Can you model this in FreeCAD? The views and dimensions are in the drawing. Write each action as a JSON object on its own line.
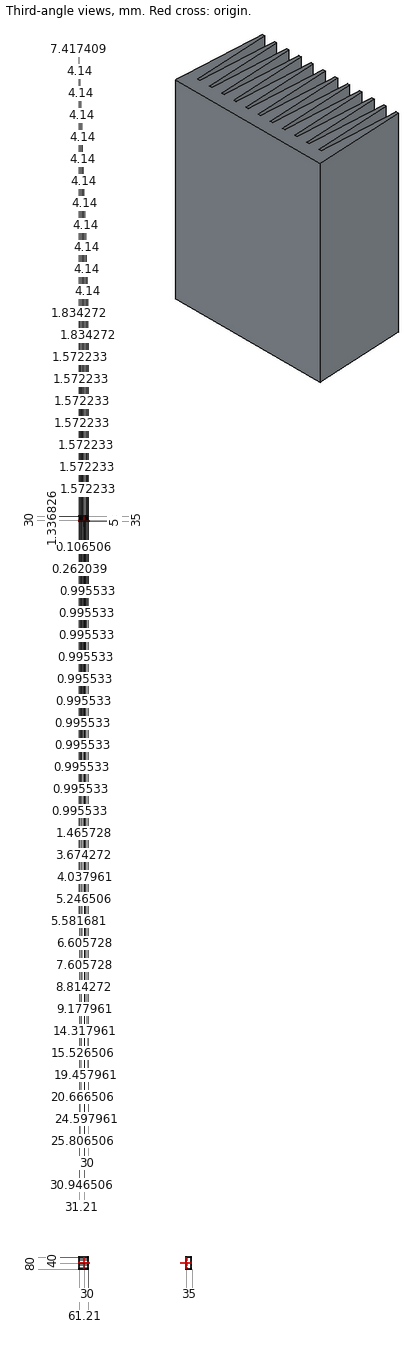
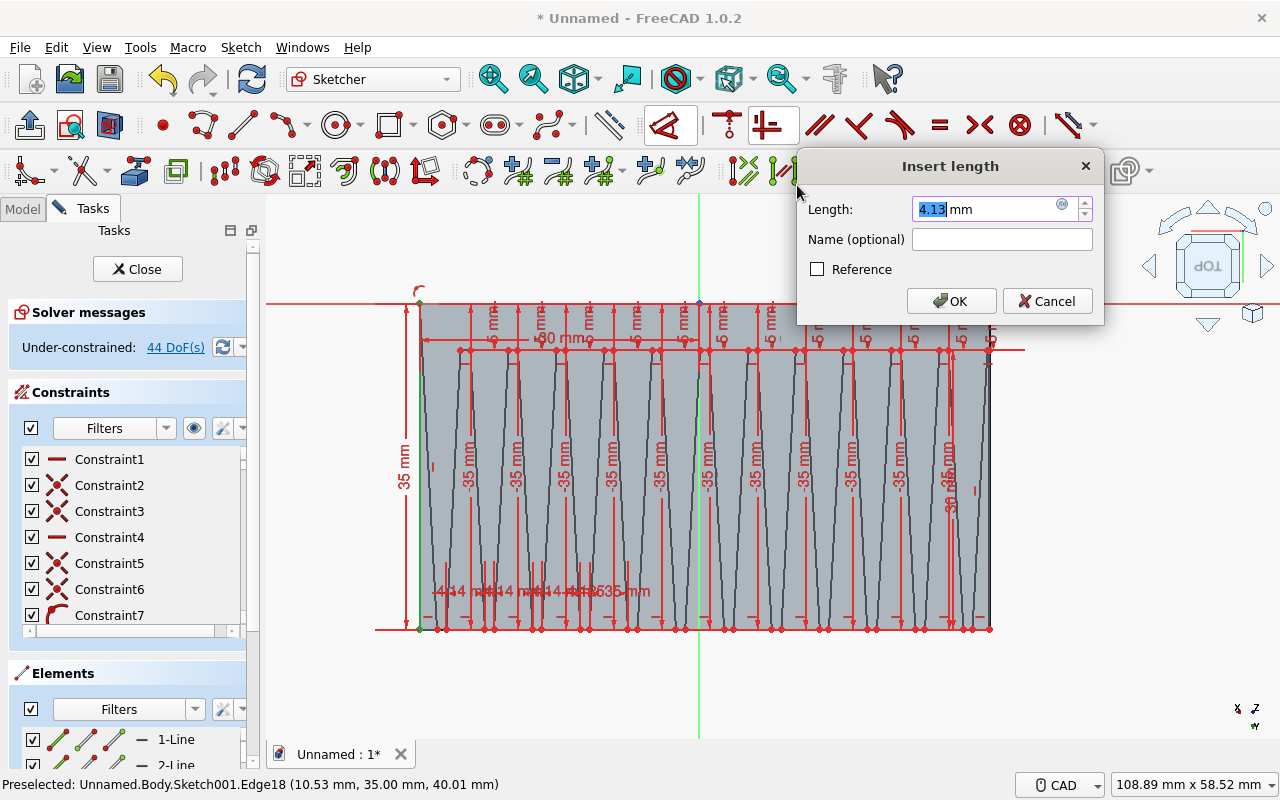
{"action": "type", "text": "4.14"}
{"action": "key", "text": "Return"}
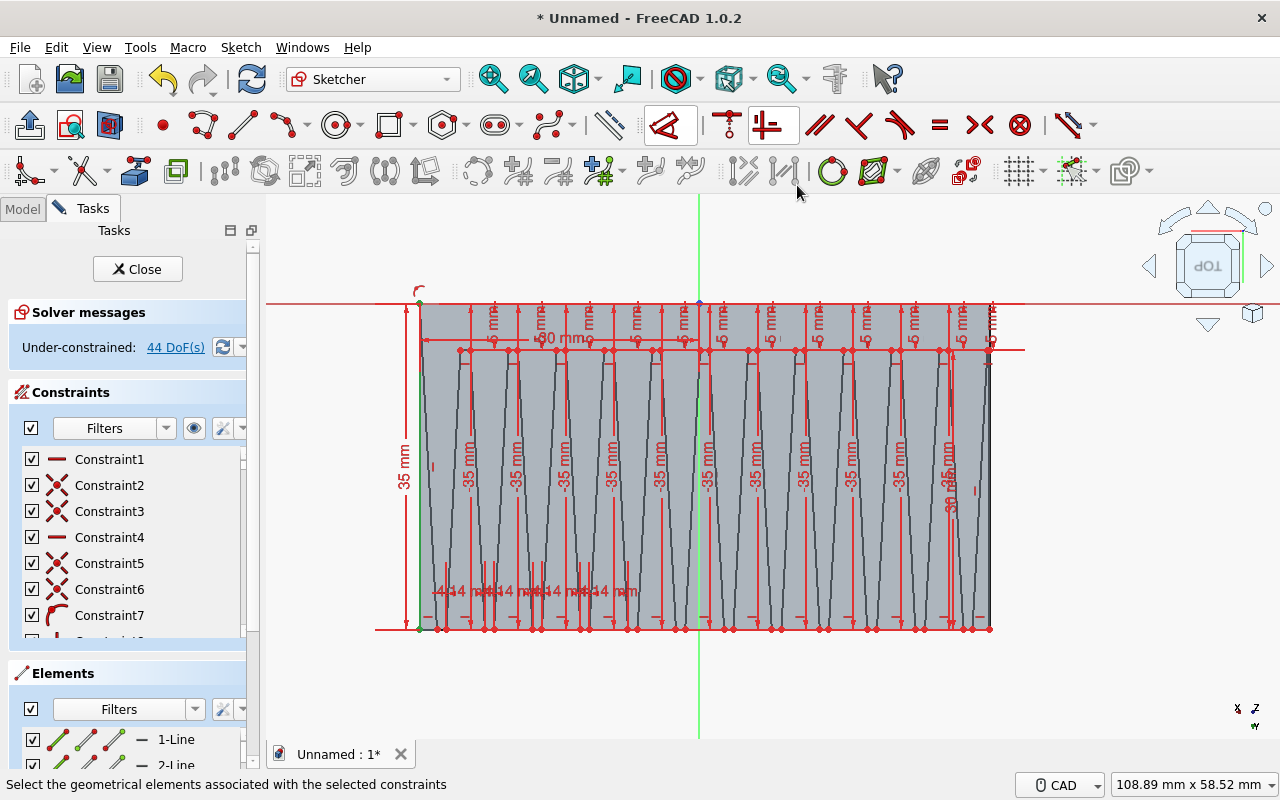
{"action": "left_click", "coordinate": [649, 630]}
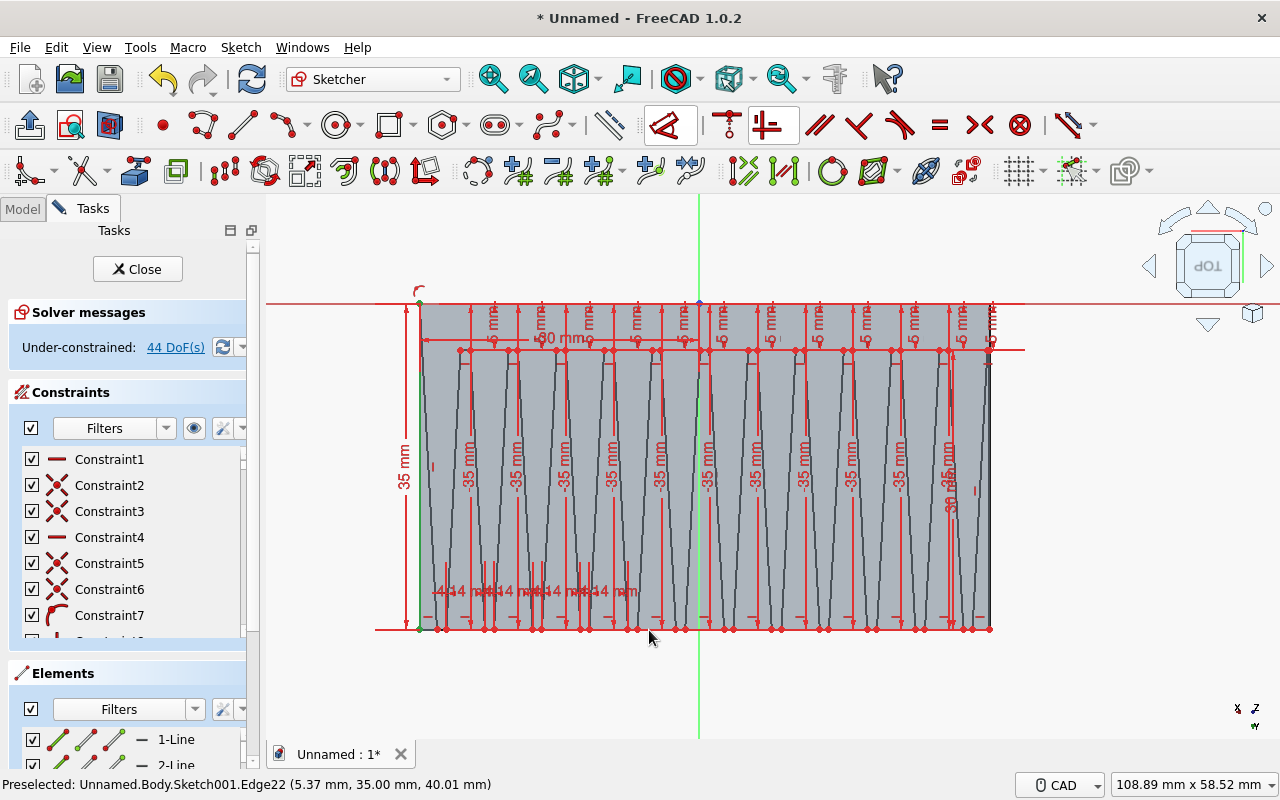
{"action": "key", "text": "l"}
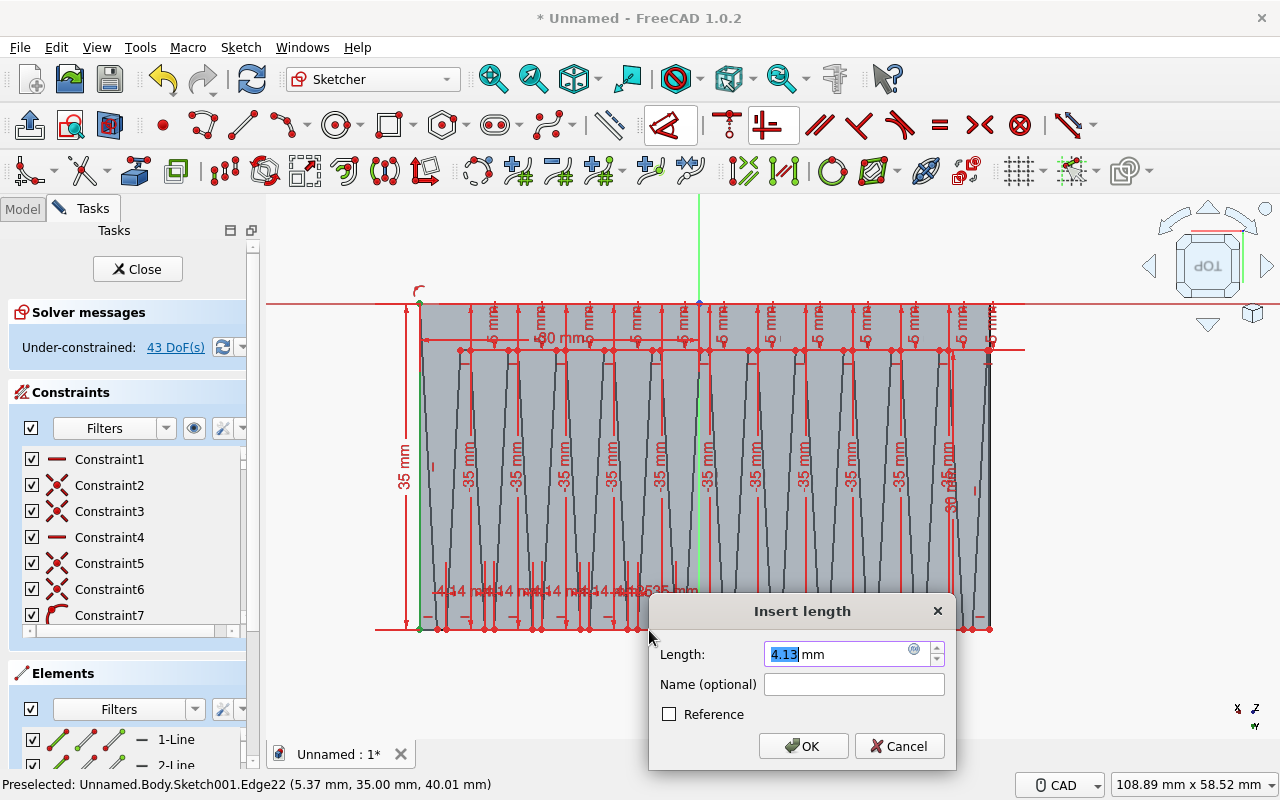
{"action": "type", "text": "4.14"}
{"action": "key", "text": "Return"}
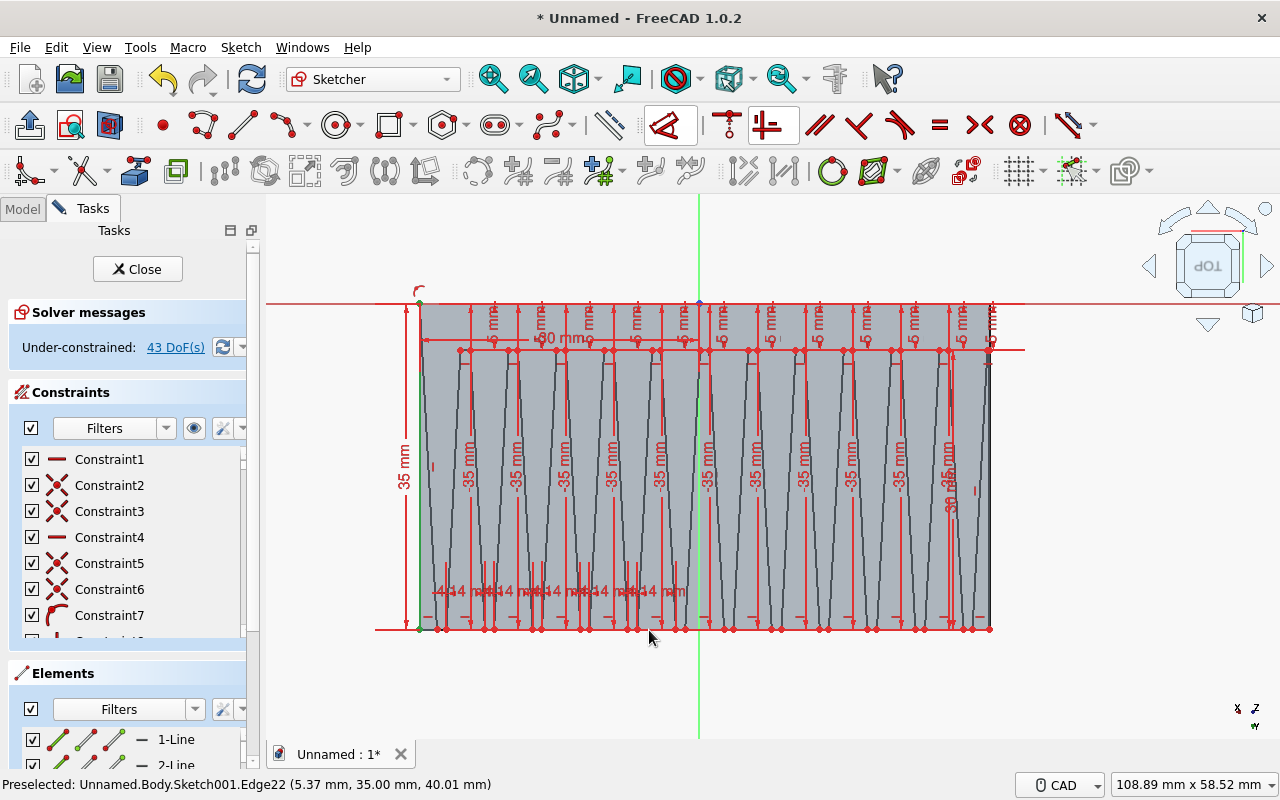
{"action": "left_click", "coordinate": [697, 630]}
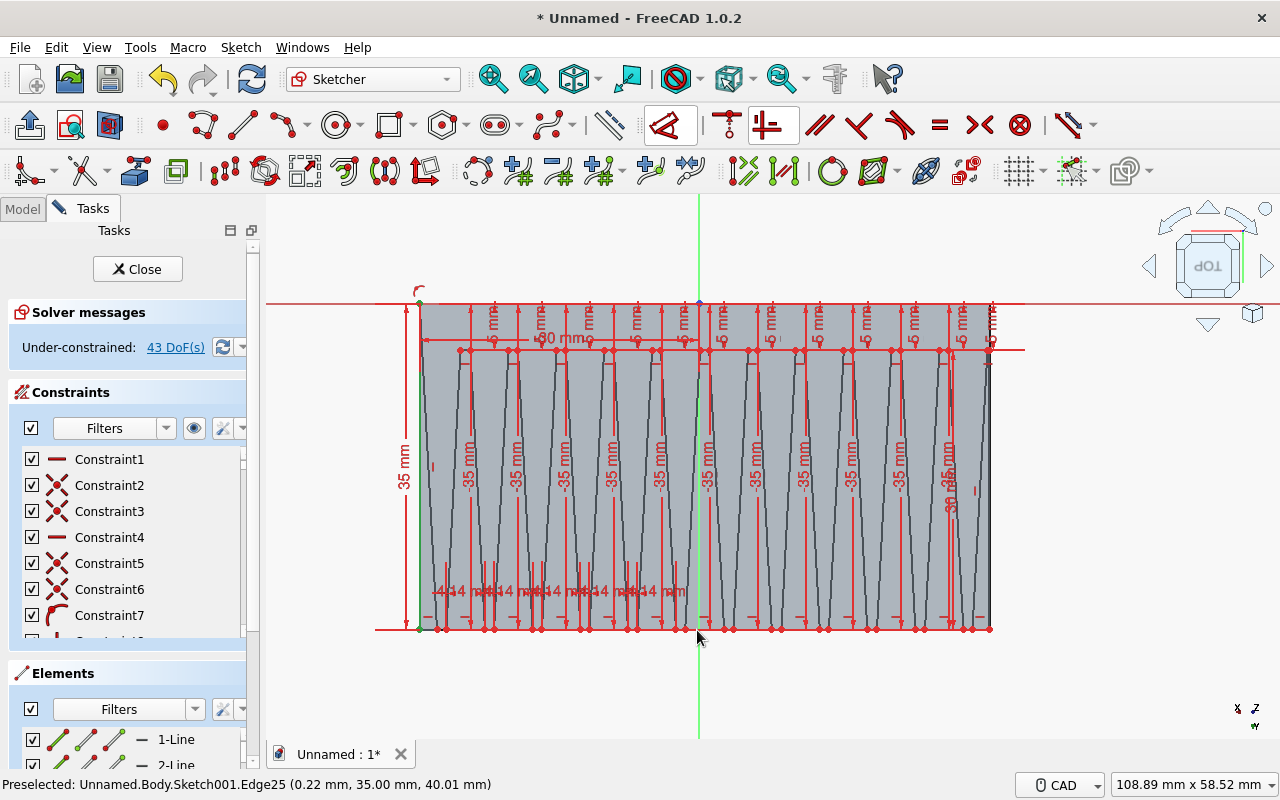
{"action": "left_click", "coordinate": [692, 126]}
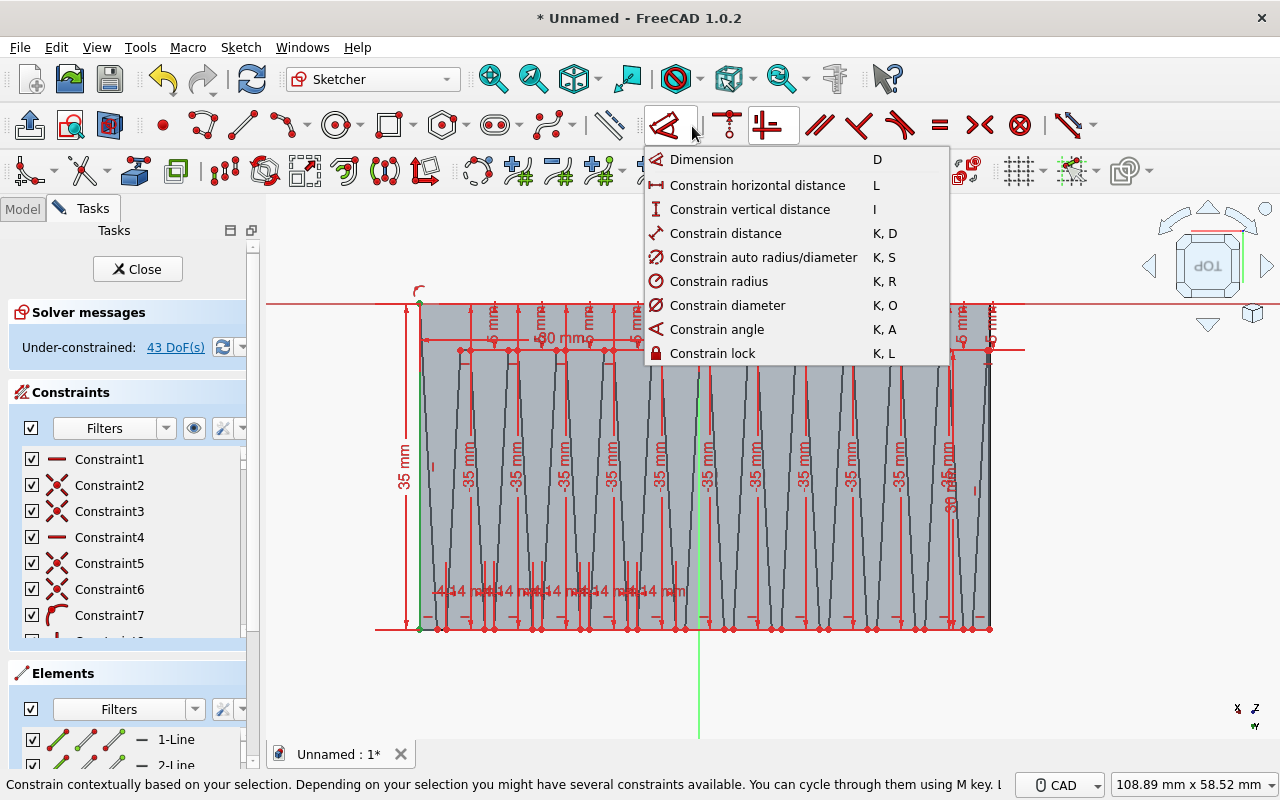
{"action": "left_click", "coordinate": [797, 185]}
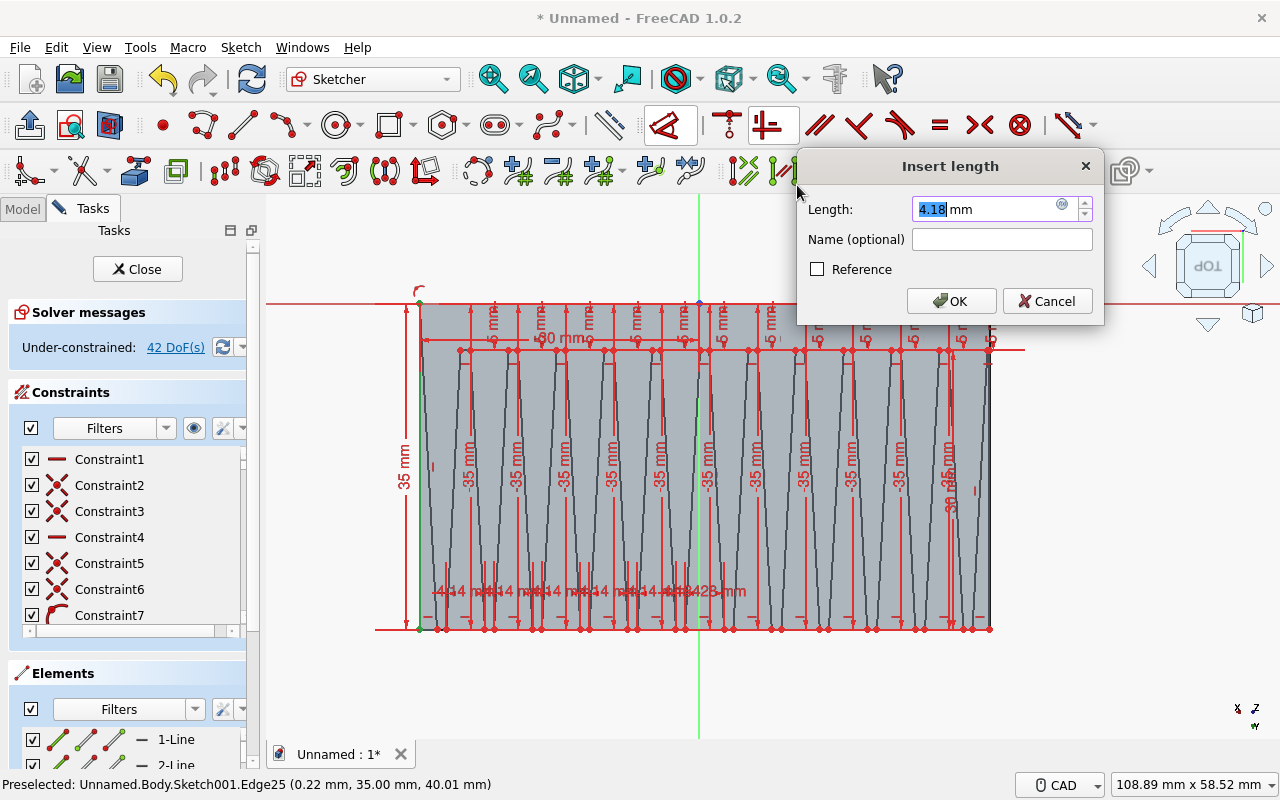
{"action": "type", "text": "4.14"}
{"action": "key", "text": "Return"}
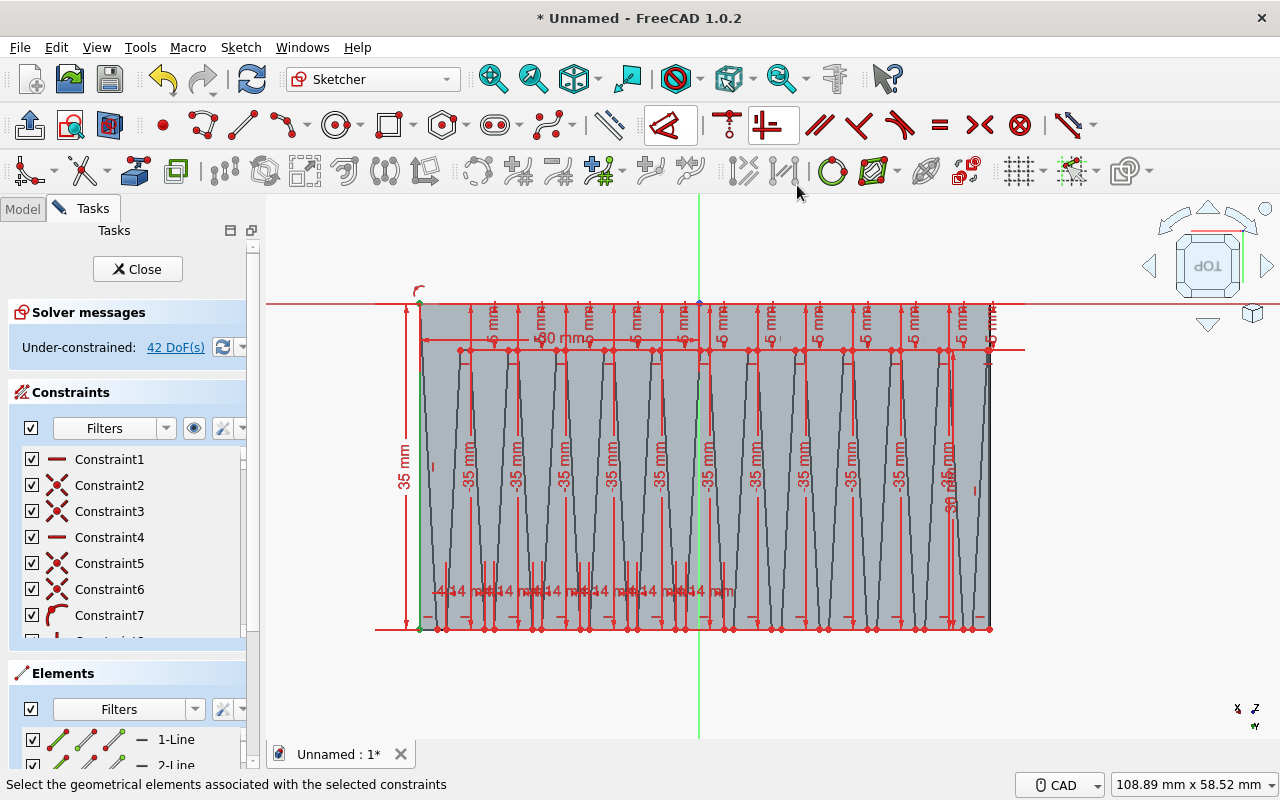
{"action": "left_click", "coordinate": [745, 630]}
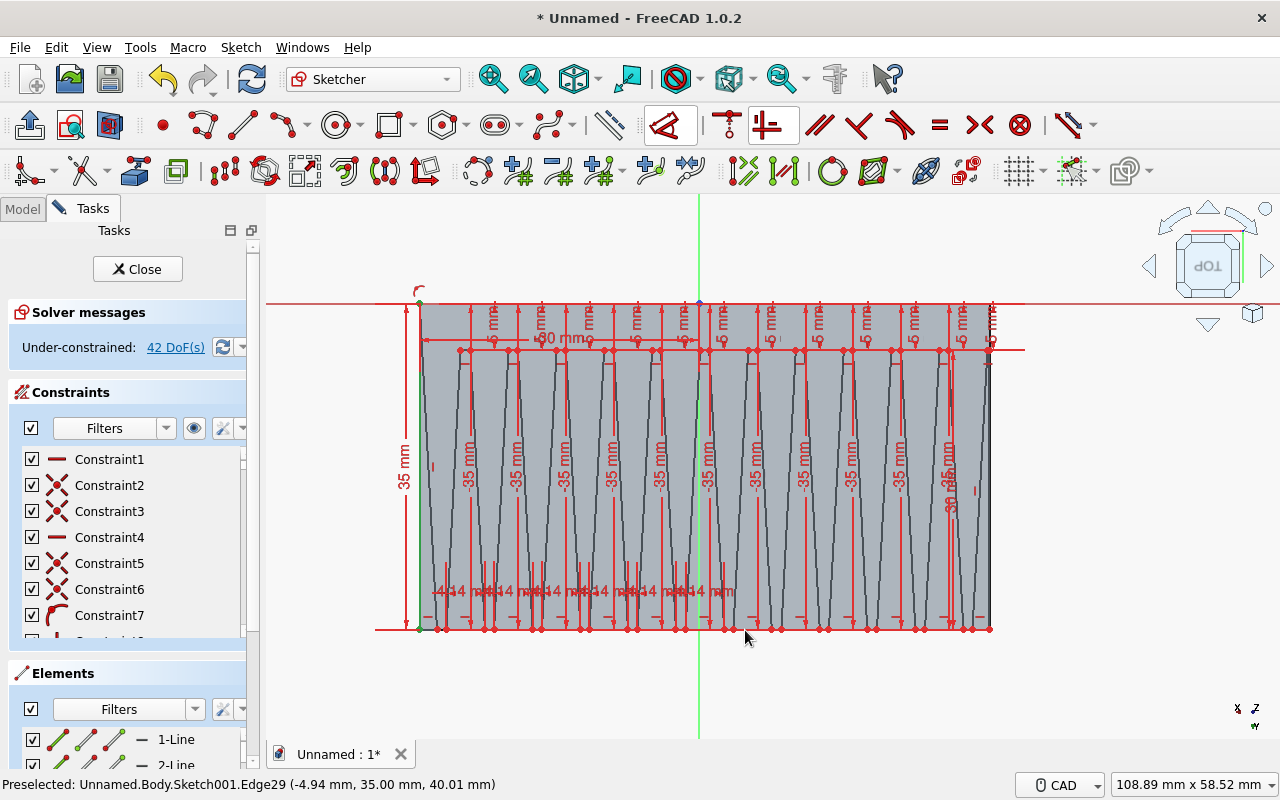
{"action": "left_click", "coordinate": [692, 126]}